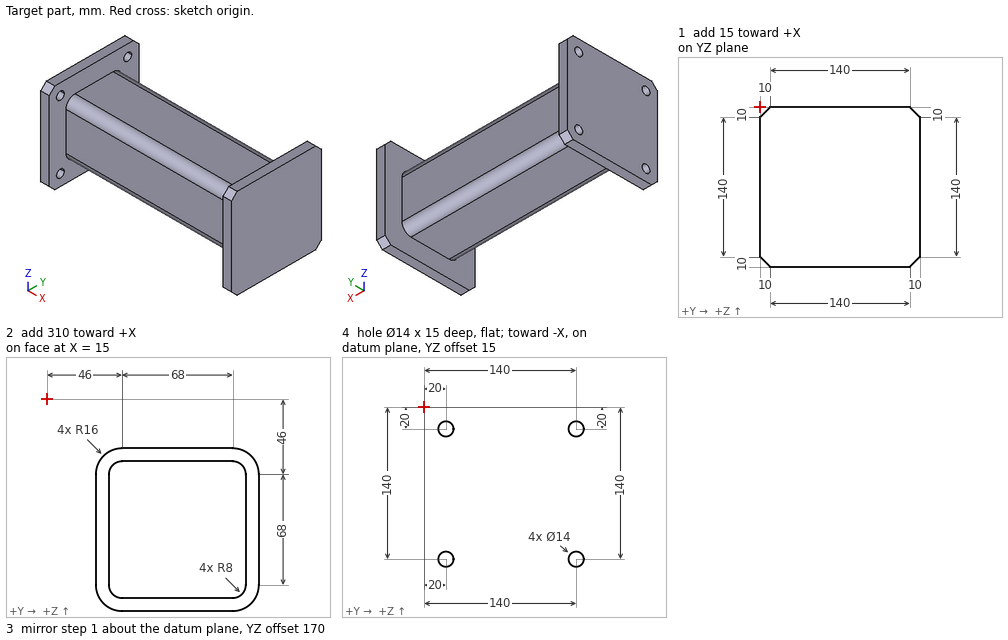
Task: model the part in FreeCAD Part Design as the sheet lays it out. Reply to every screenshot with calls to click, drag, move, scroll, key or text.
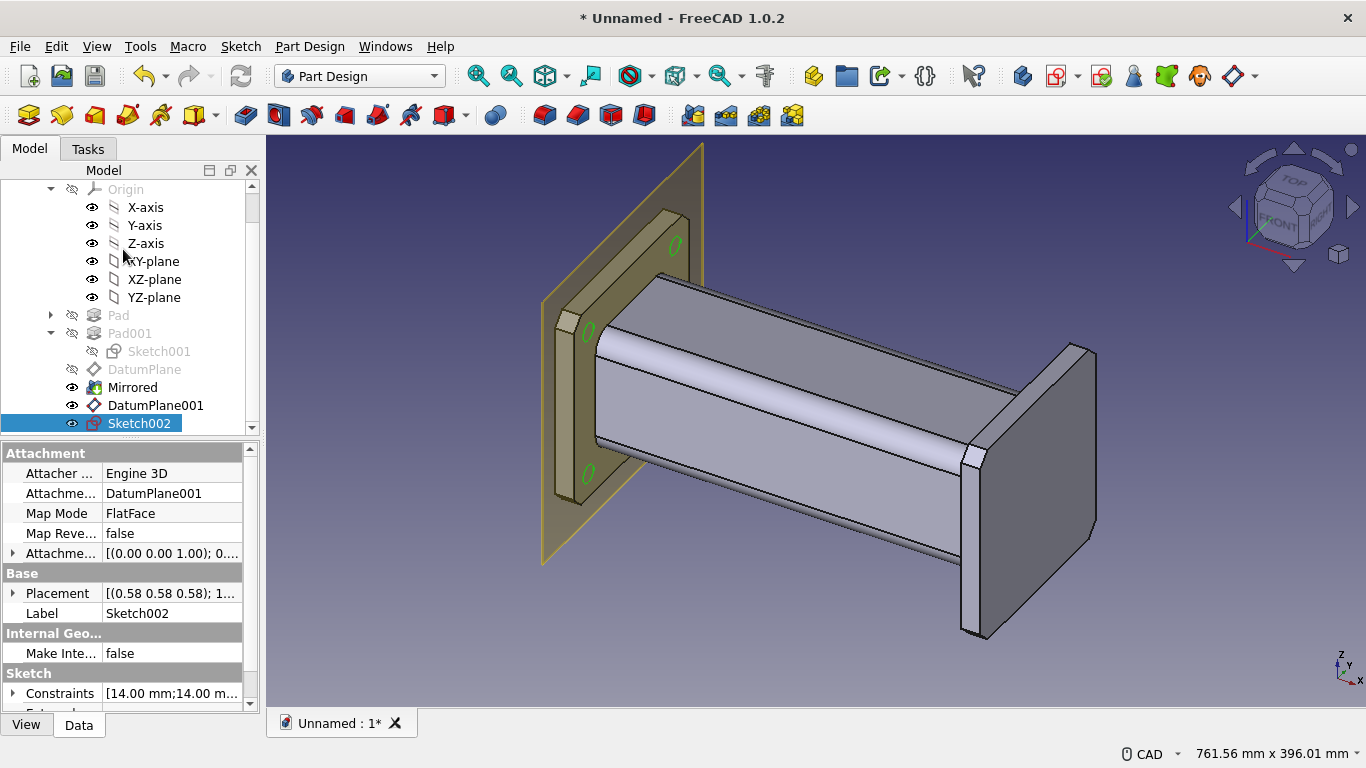
click(279, 116)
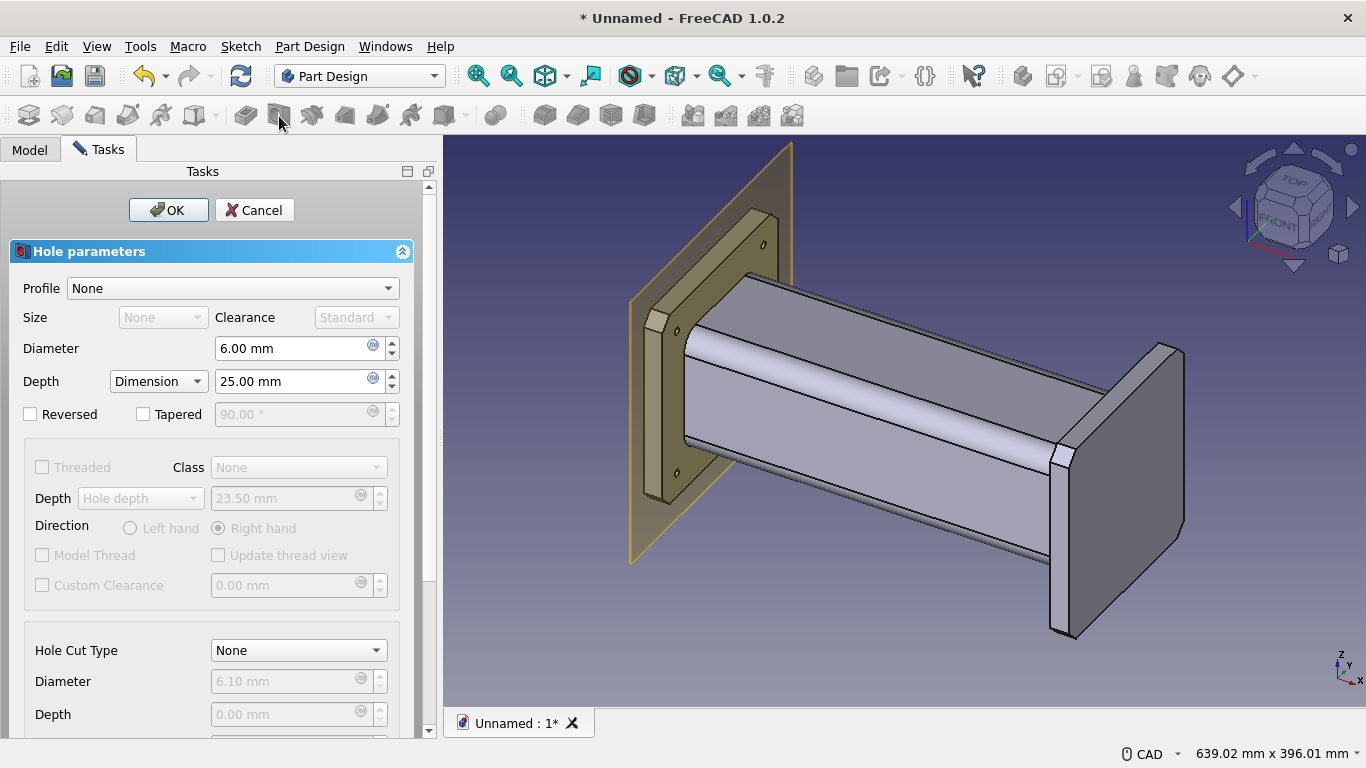
triple_click(300, 348)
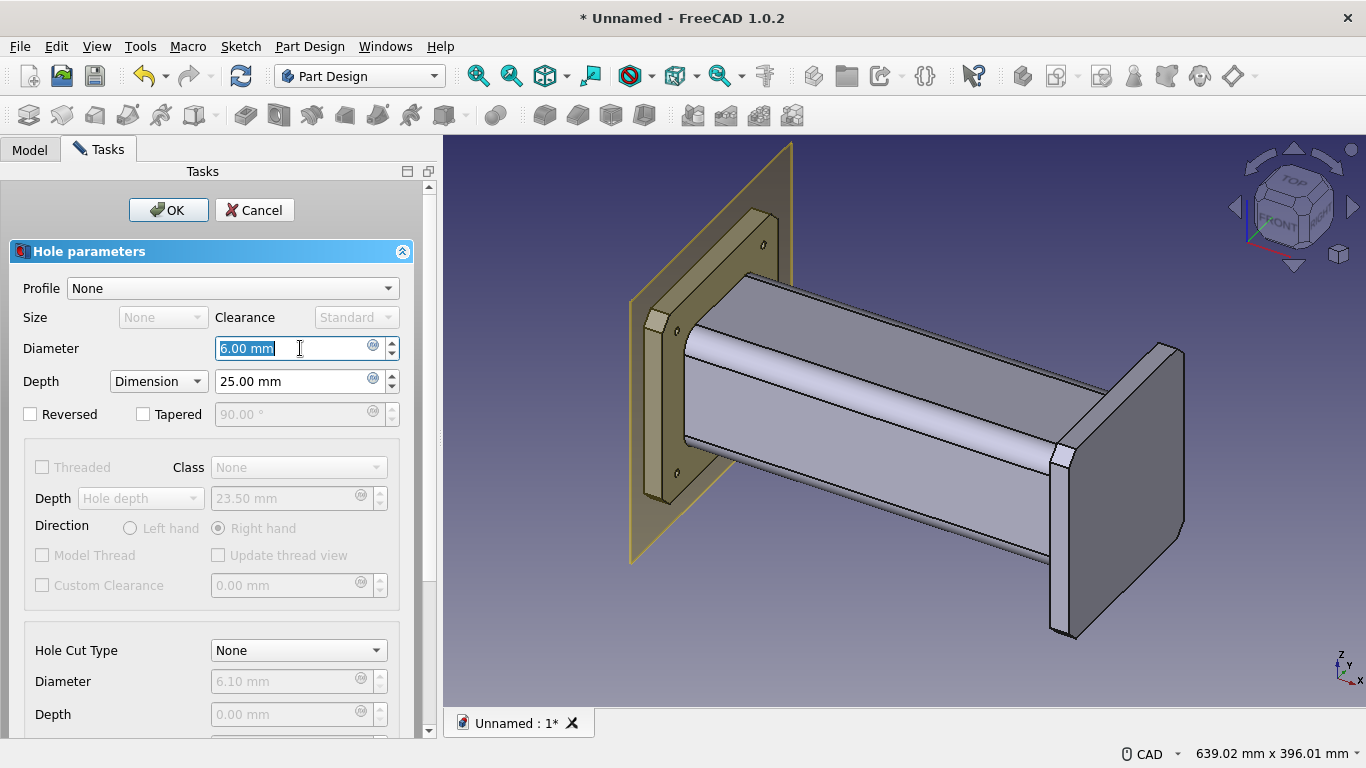
text(14)
key(Tab)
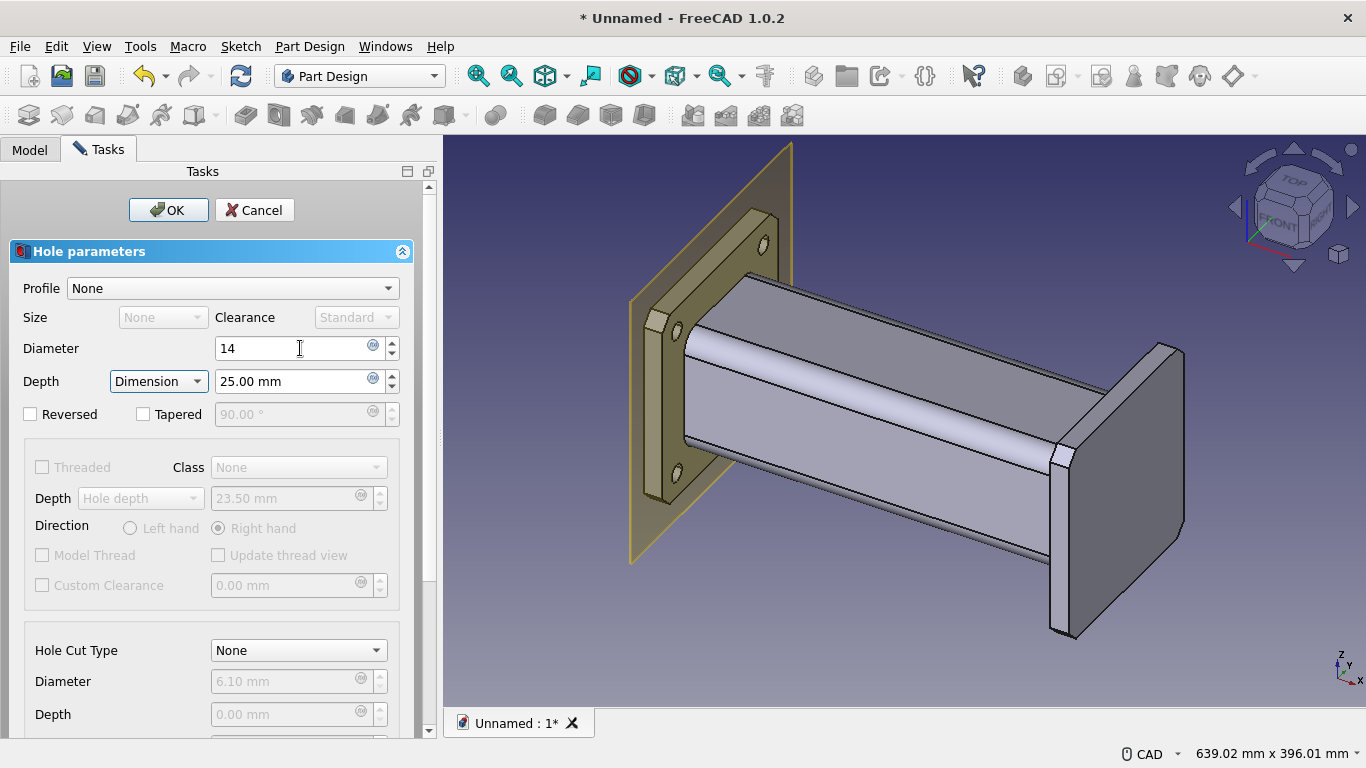
triple_click(300, 382)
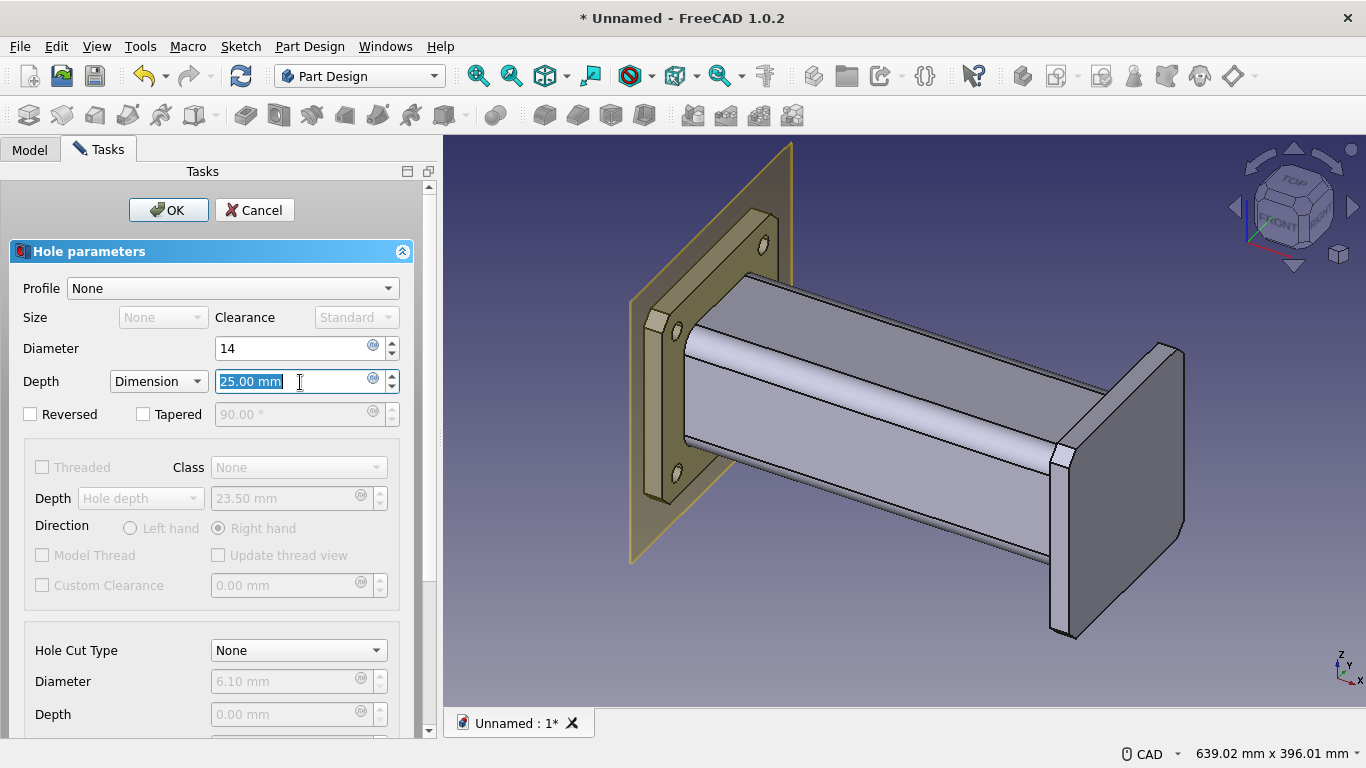
text(15)
key(Tab)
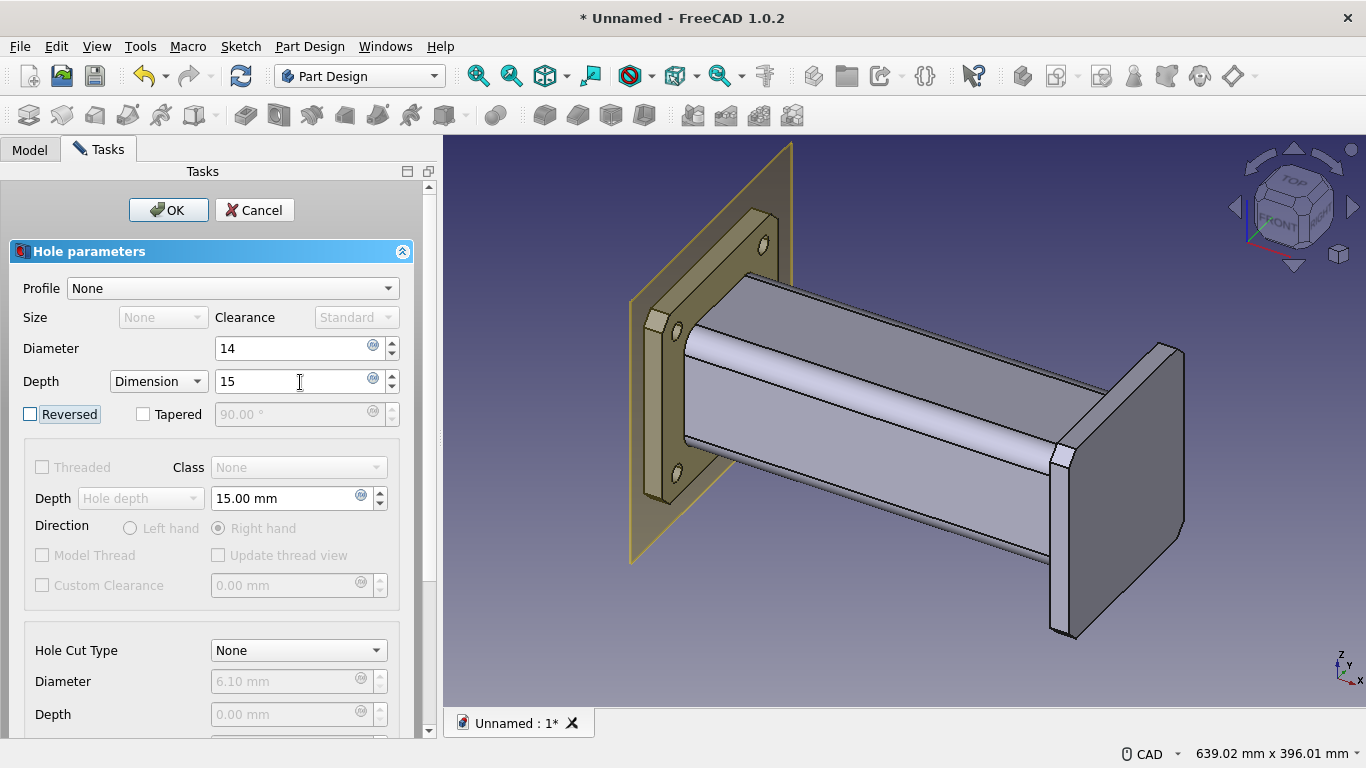
scroll(429, 460, down, 3)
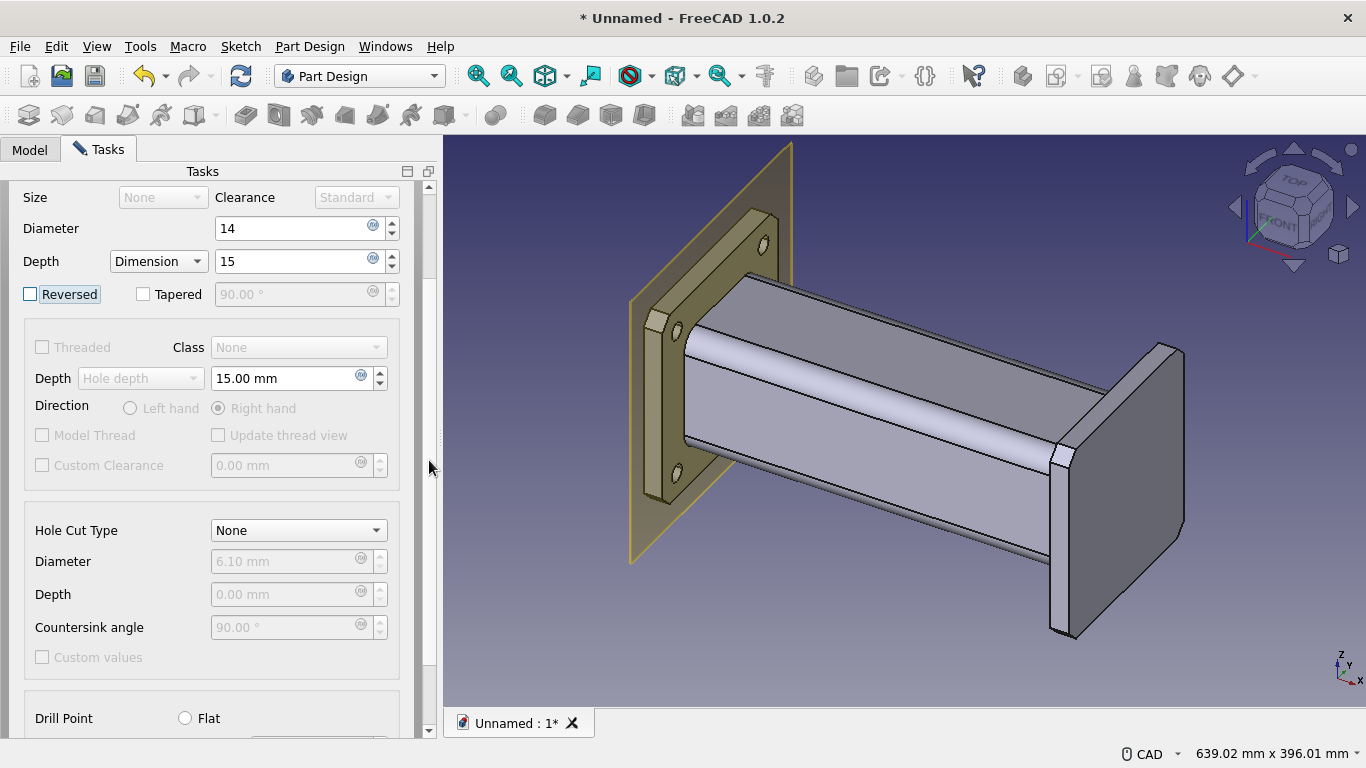
click(186, 656)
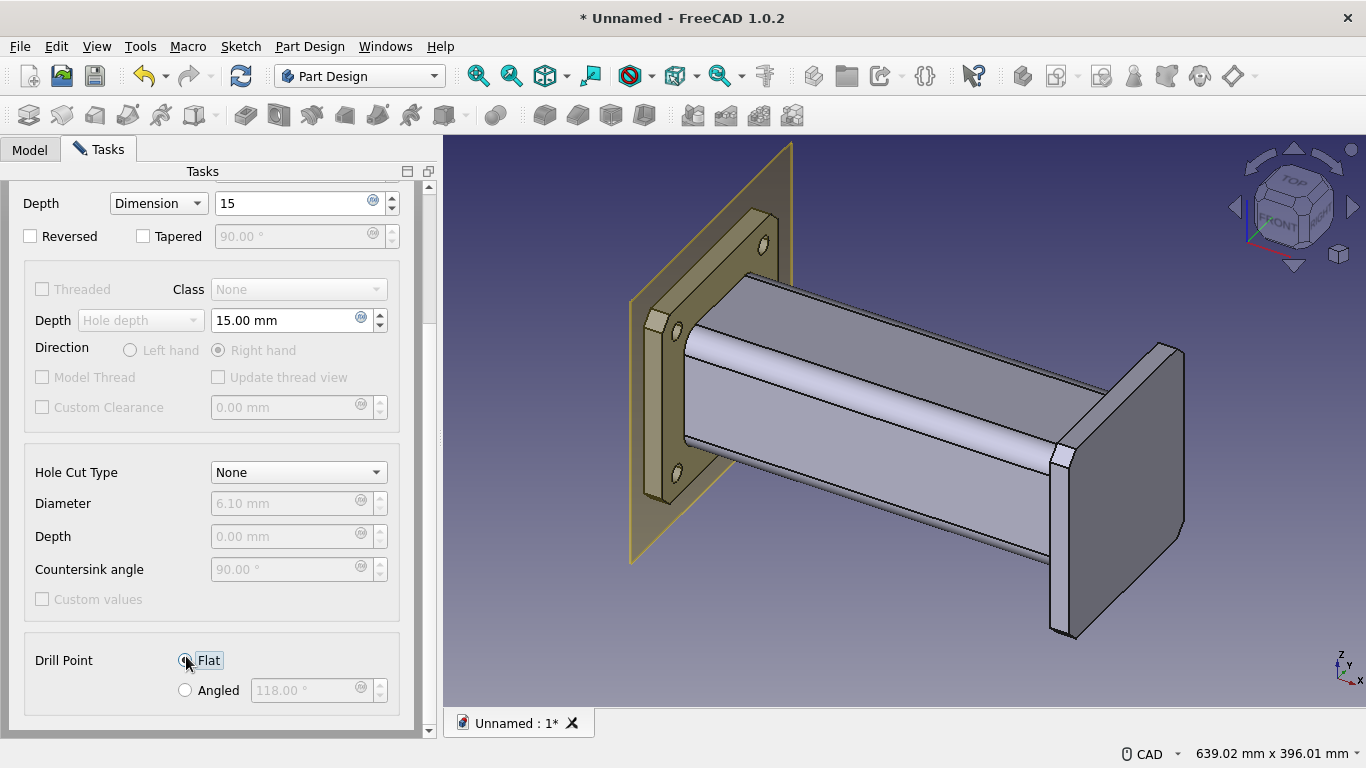
scroll(429, 460, up, 4)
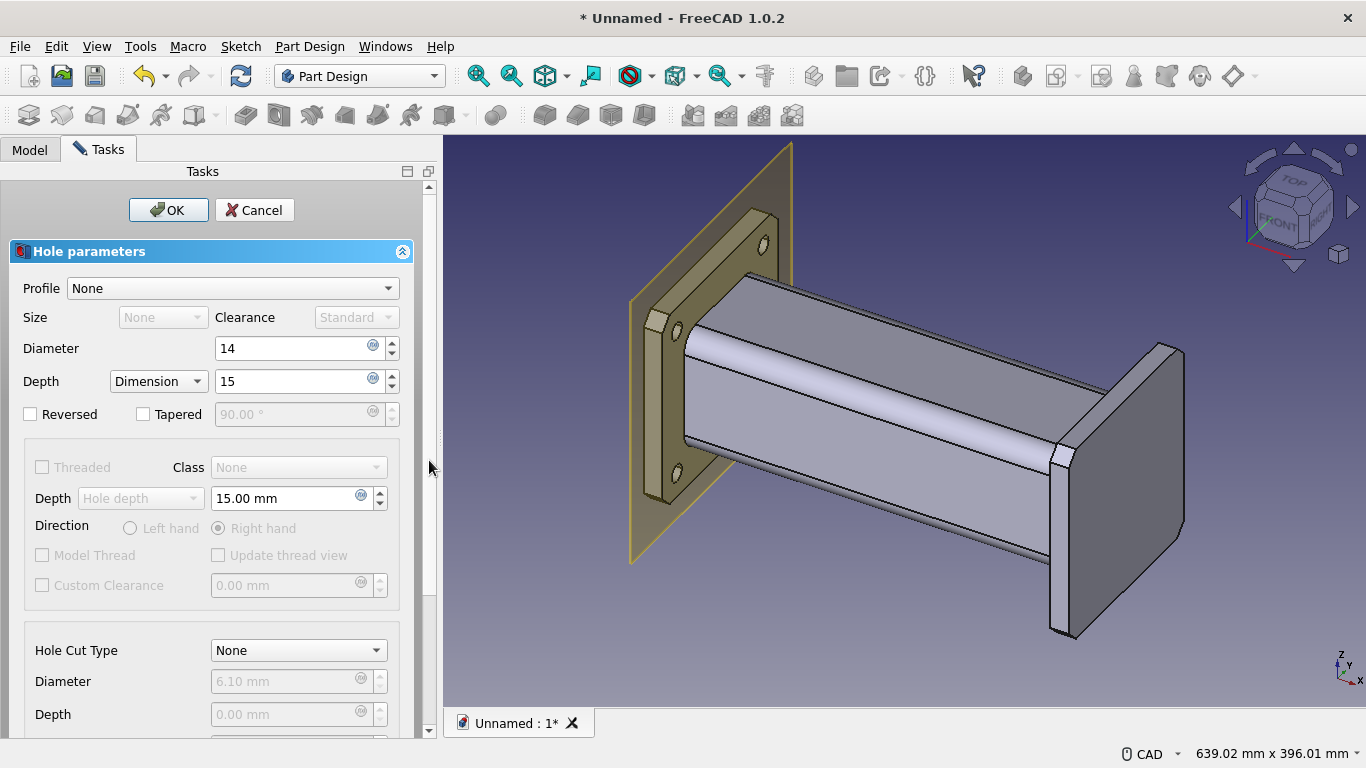
click(169, 210)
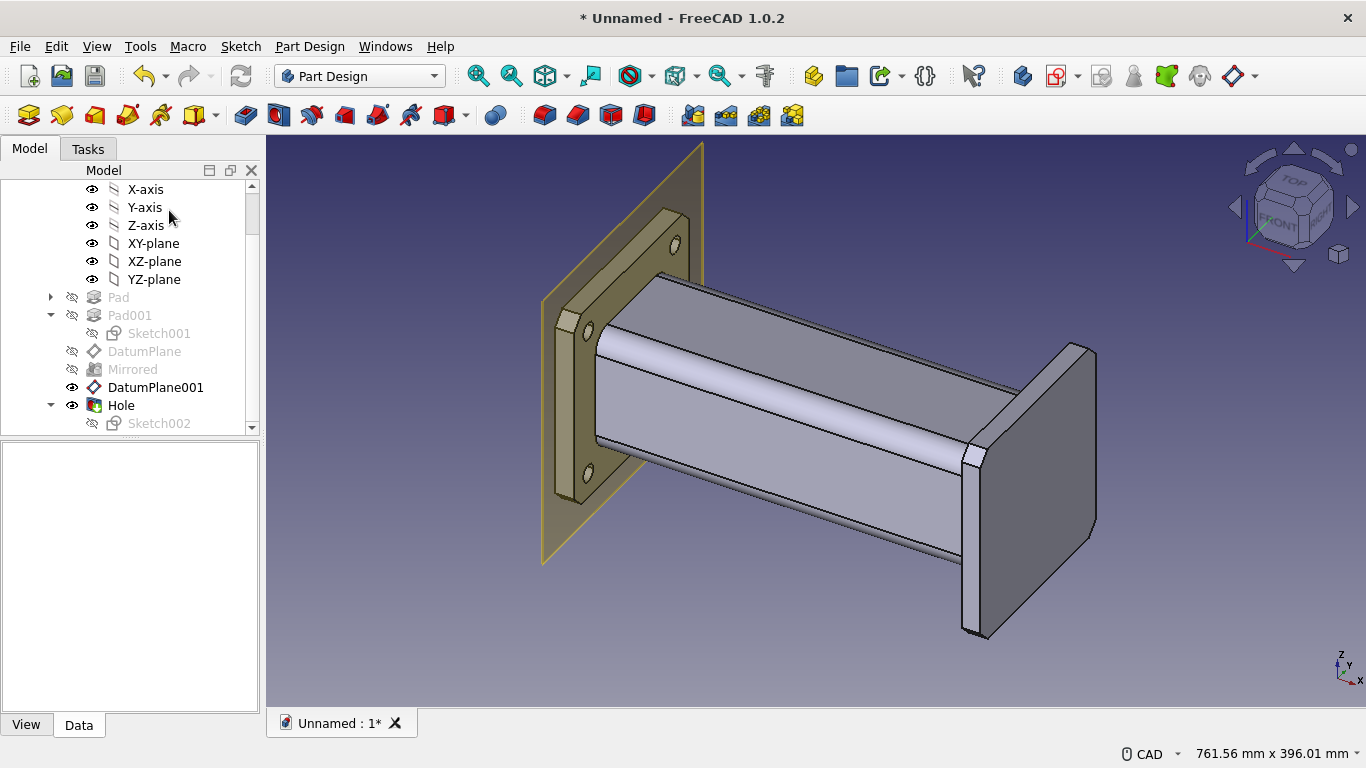
click(117, 387)
key(space)